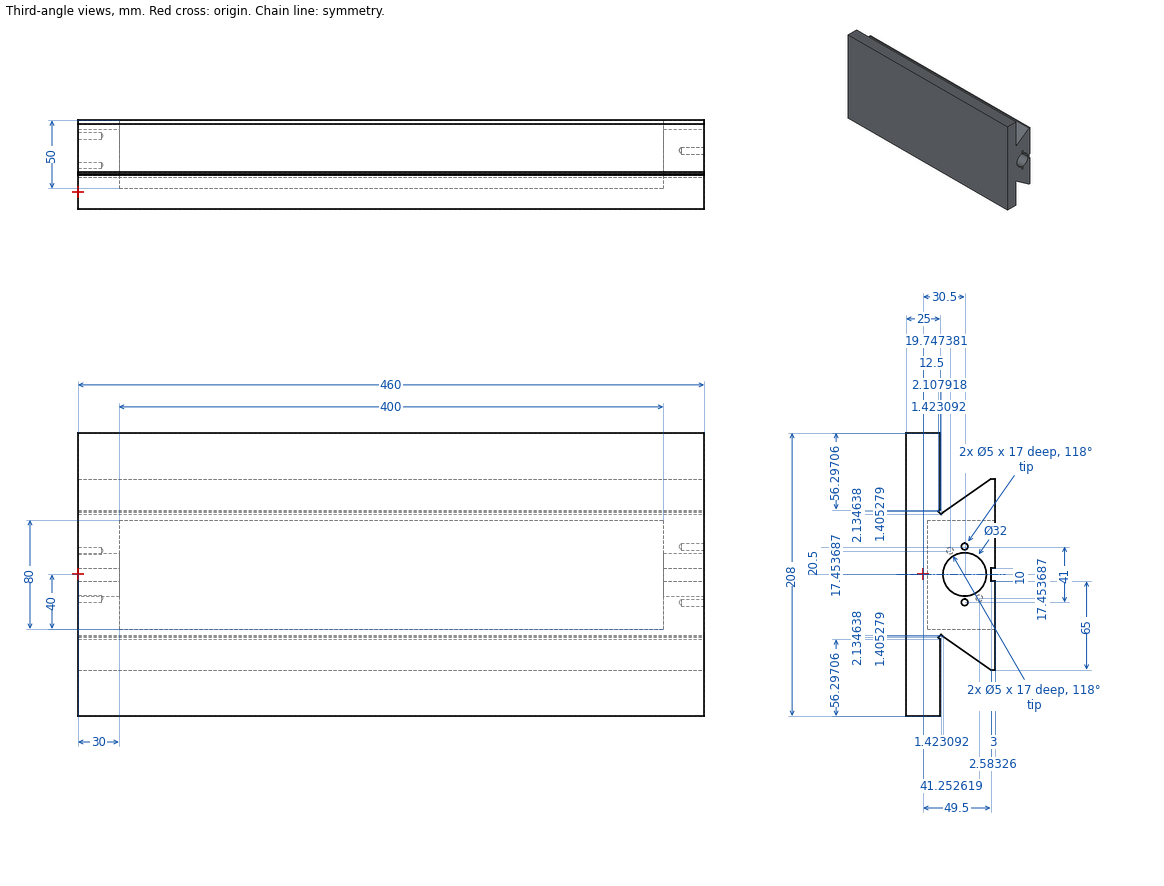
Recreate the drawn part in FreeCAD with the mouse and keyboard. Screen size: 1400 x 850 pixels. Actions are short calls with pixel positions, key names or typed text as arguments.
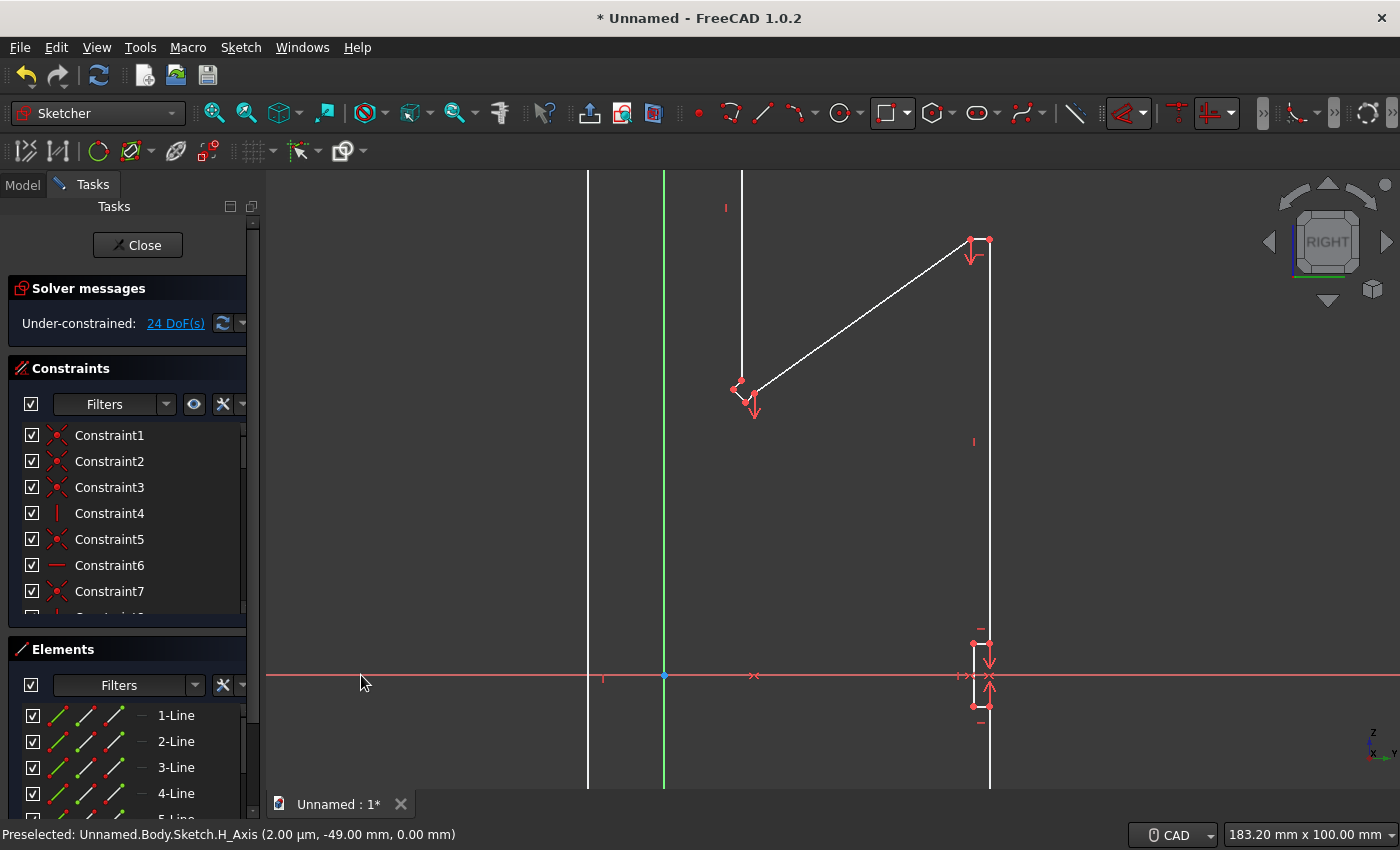
scroll(754, 395, down, 6)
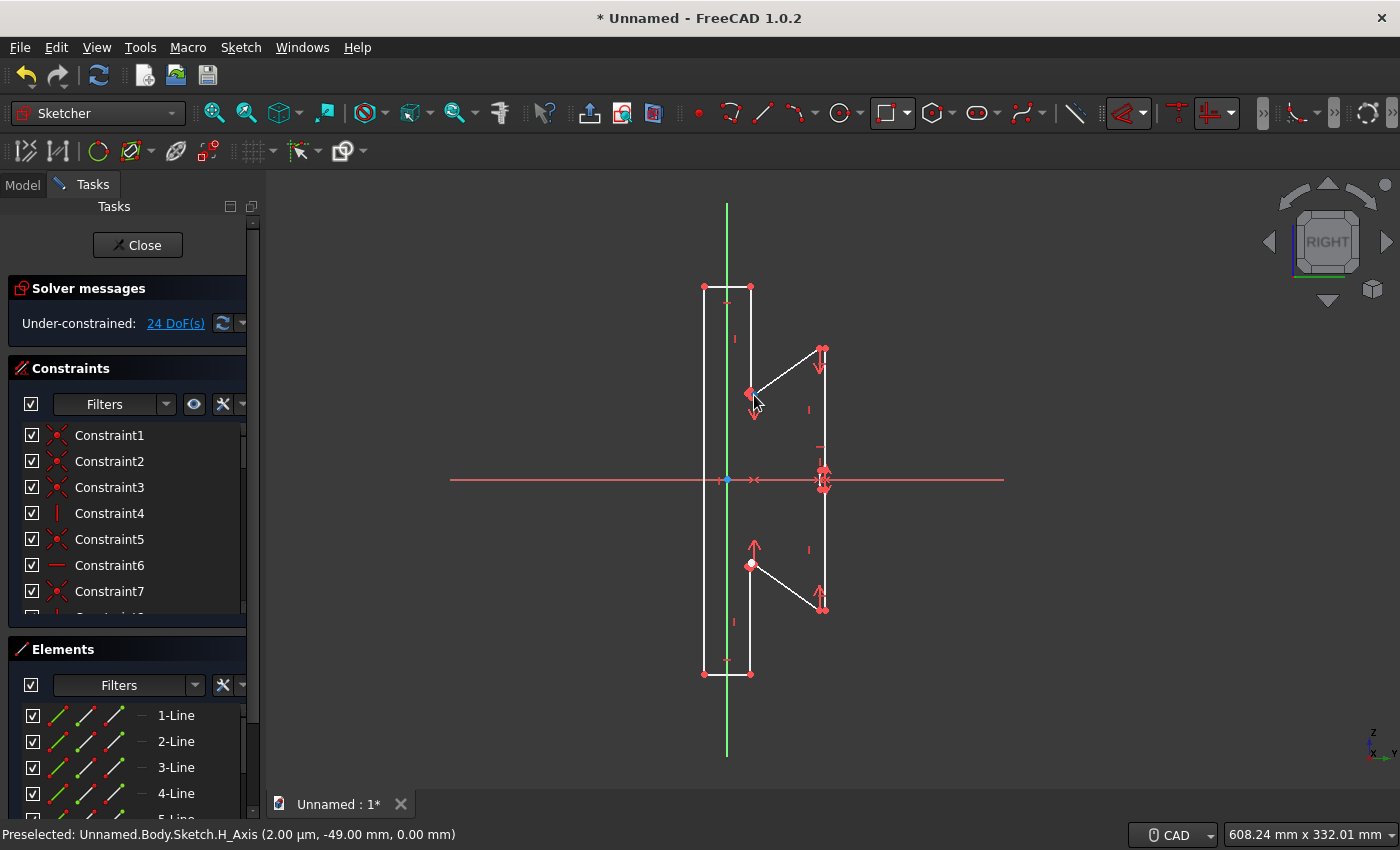
scroll(752, 563, up, 7)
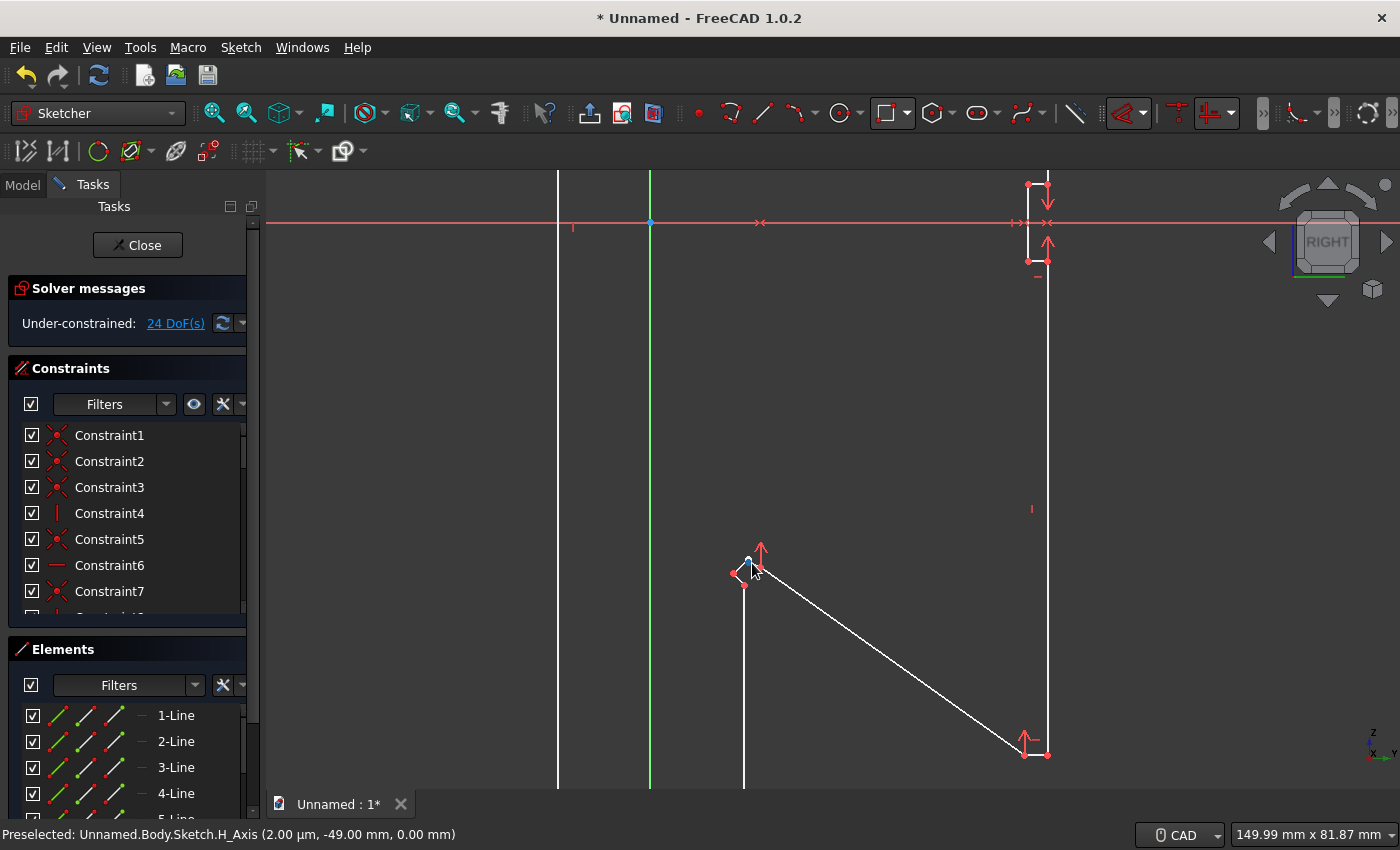
click(749, 563)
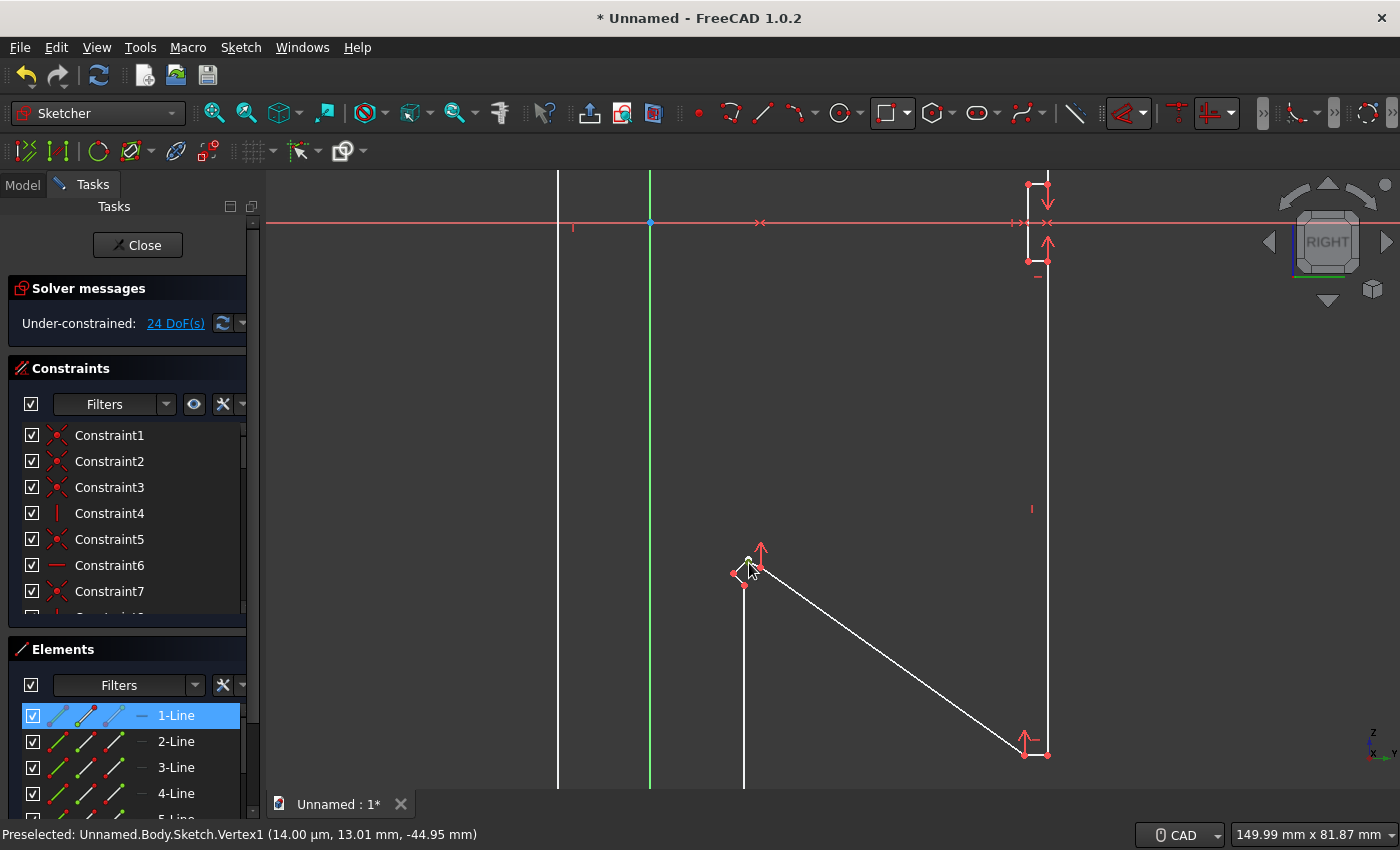
scroll(752, 563, down, 7)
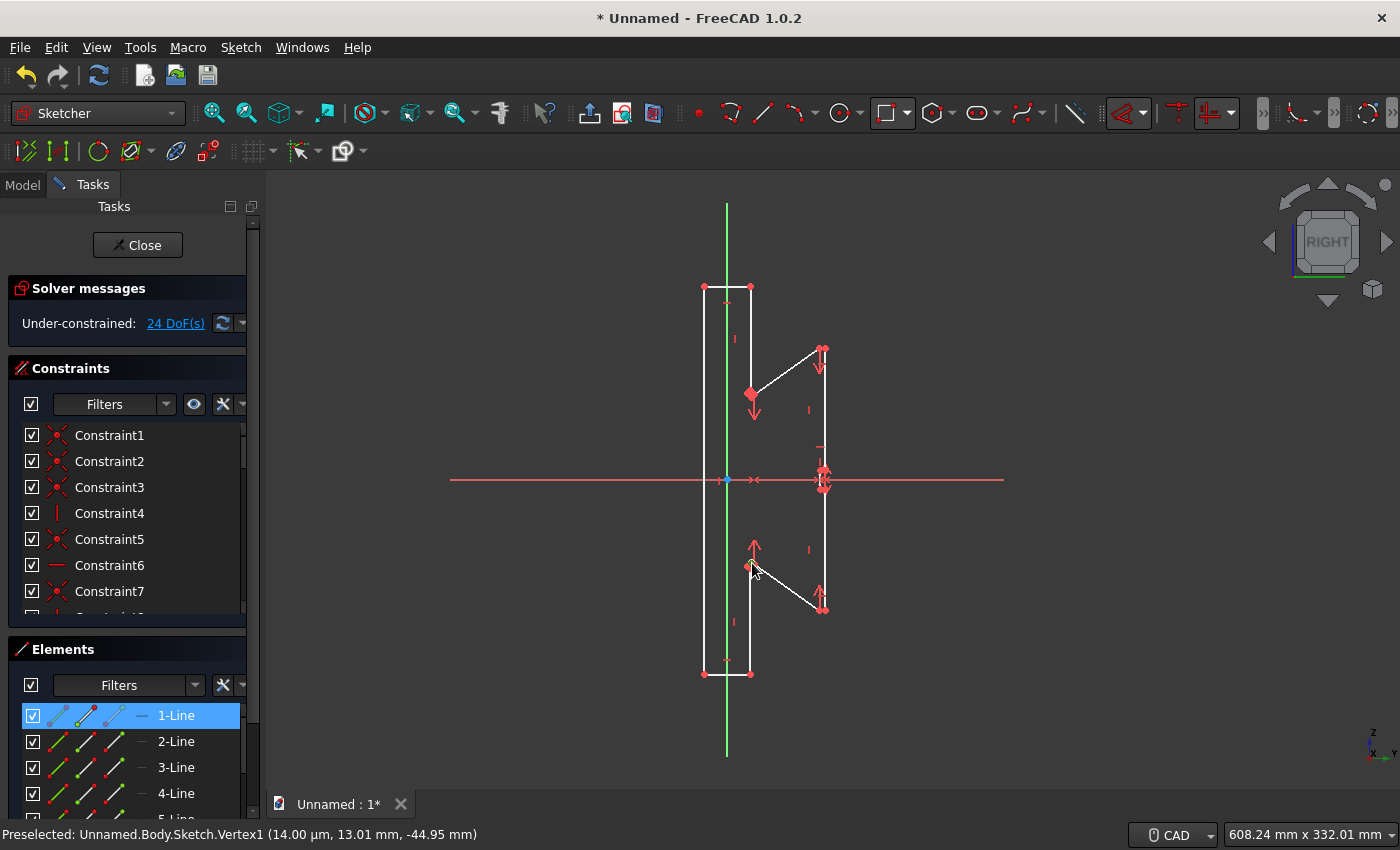
scroll(752, 398, up, 6)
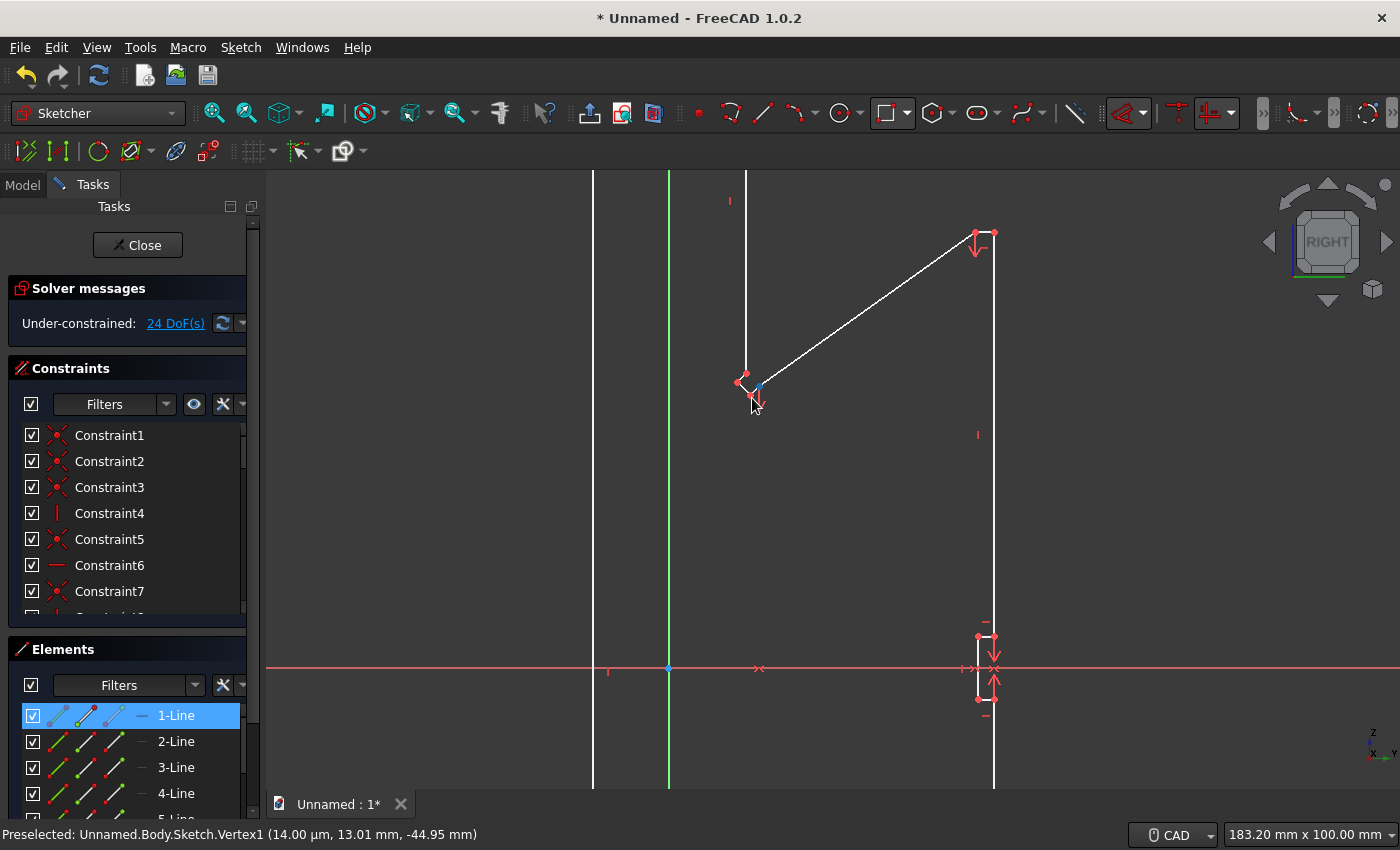
click(750, 396)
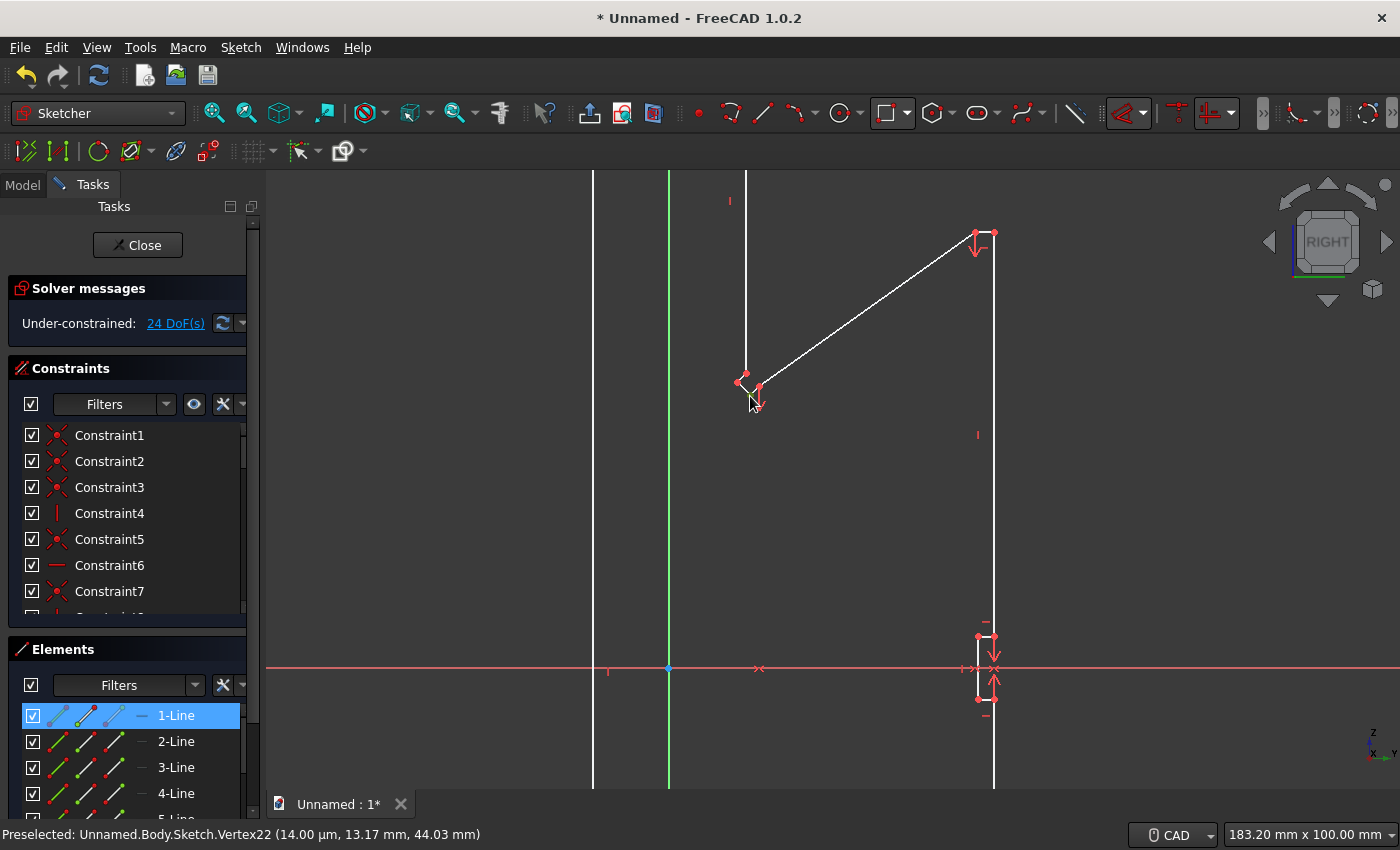
click(361, 668)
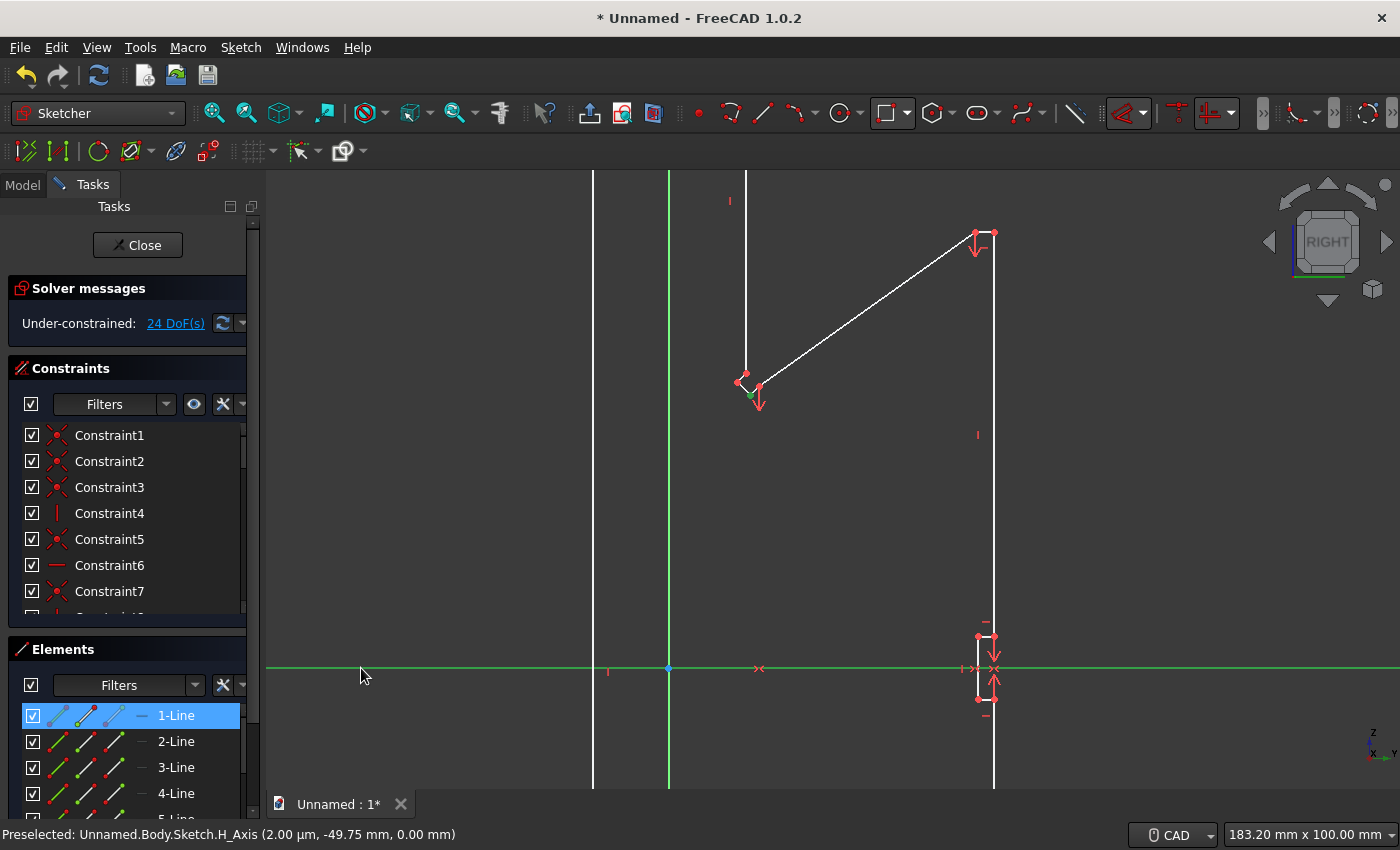
key(s)